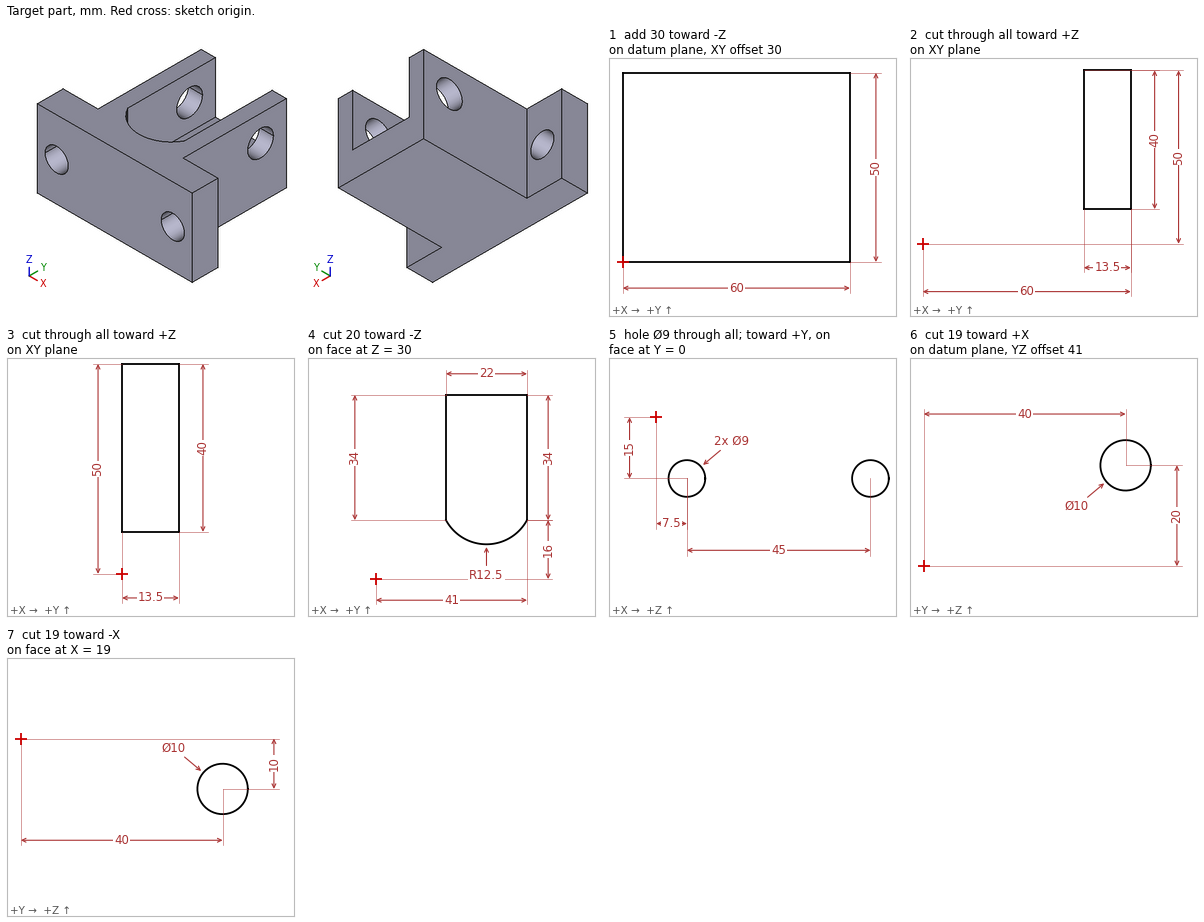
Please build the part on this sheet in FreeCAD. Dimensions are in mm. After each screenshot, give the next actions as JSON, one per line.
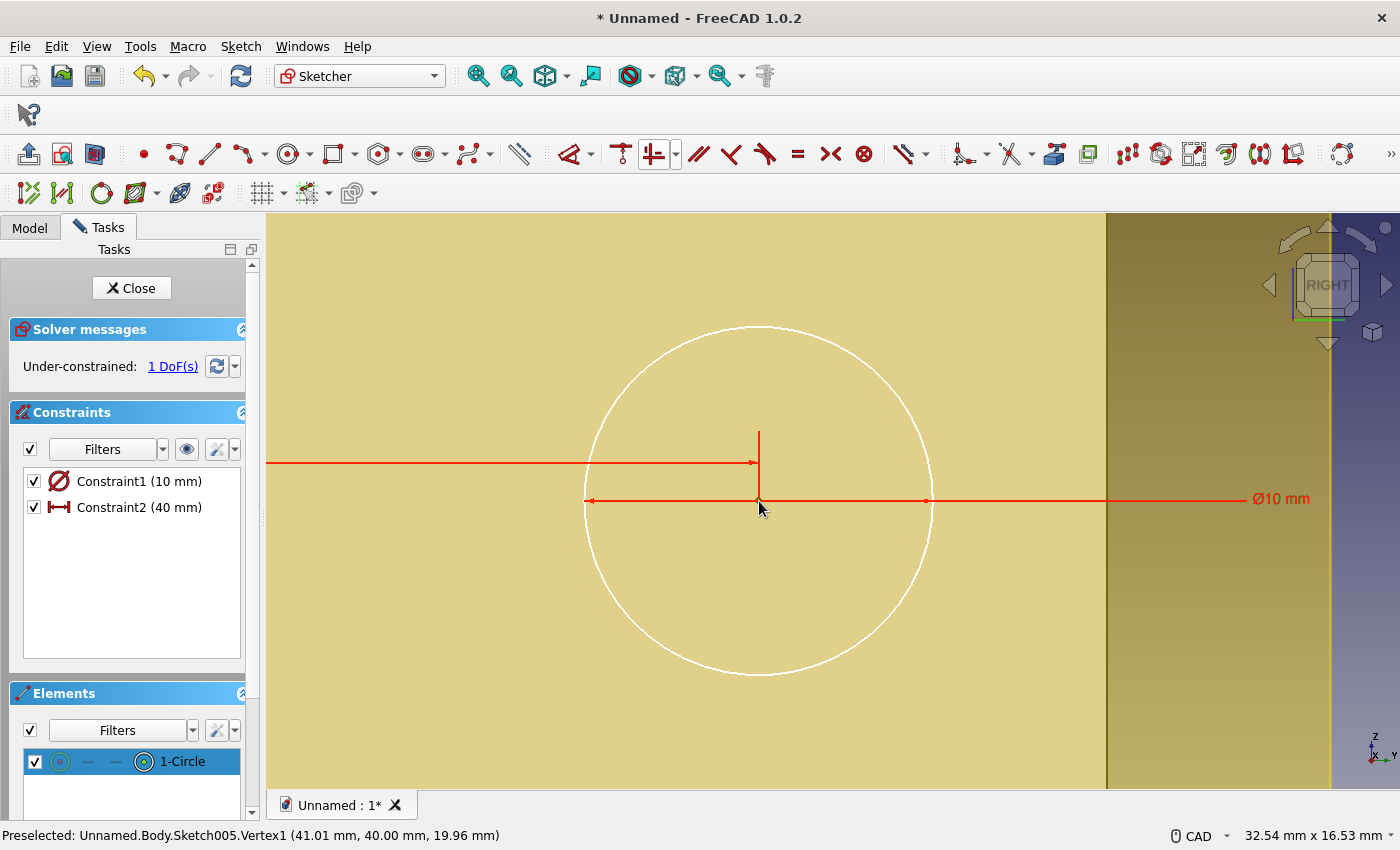
{"action": "key", "text": "i"}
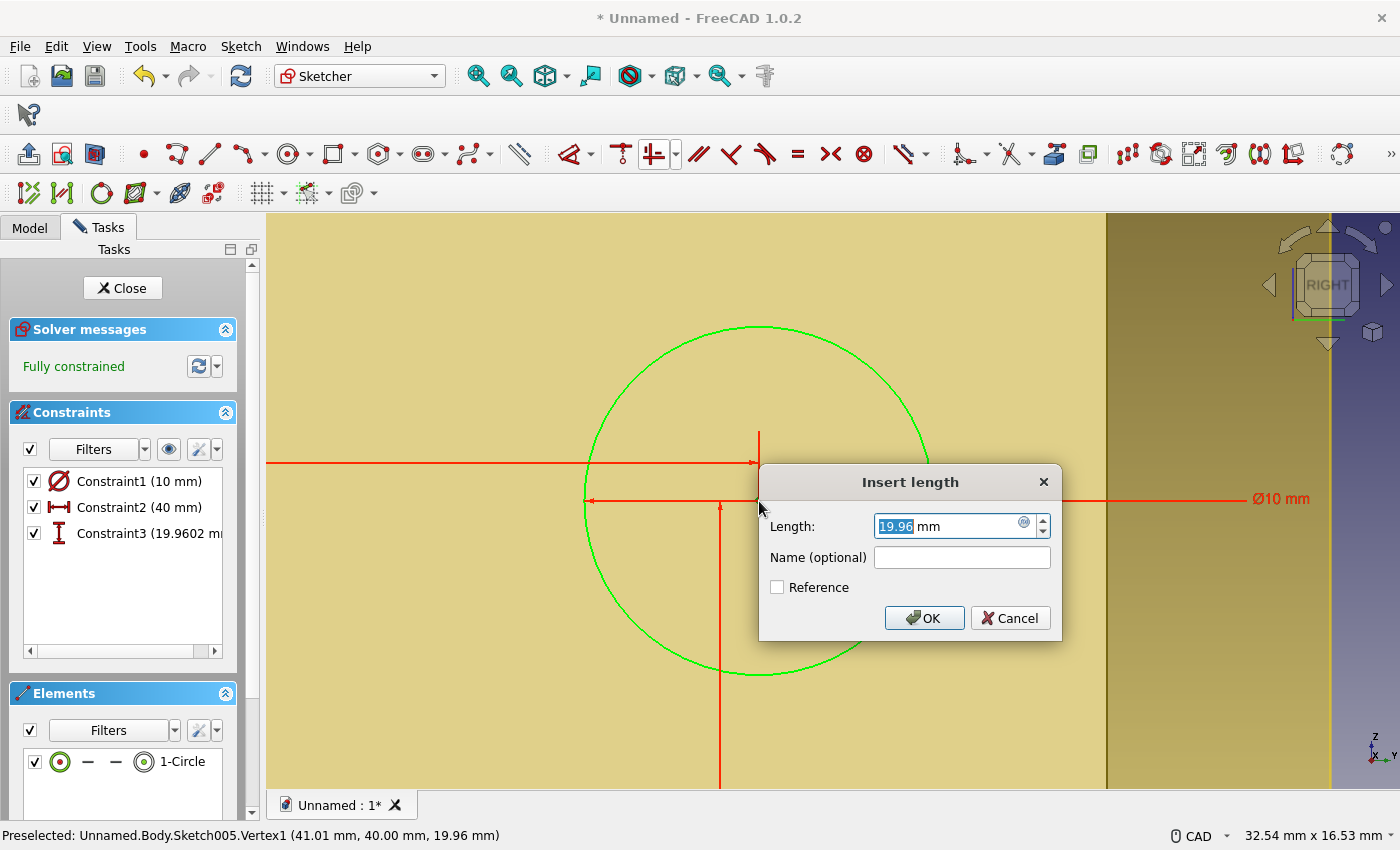
{"action": "type", "text": "20"}
{"action": "key", "text": "Return"}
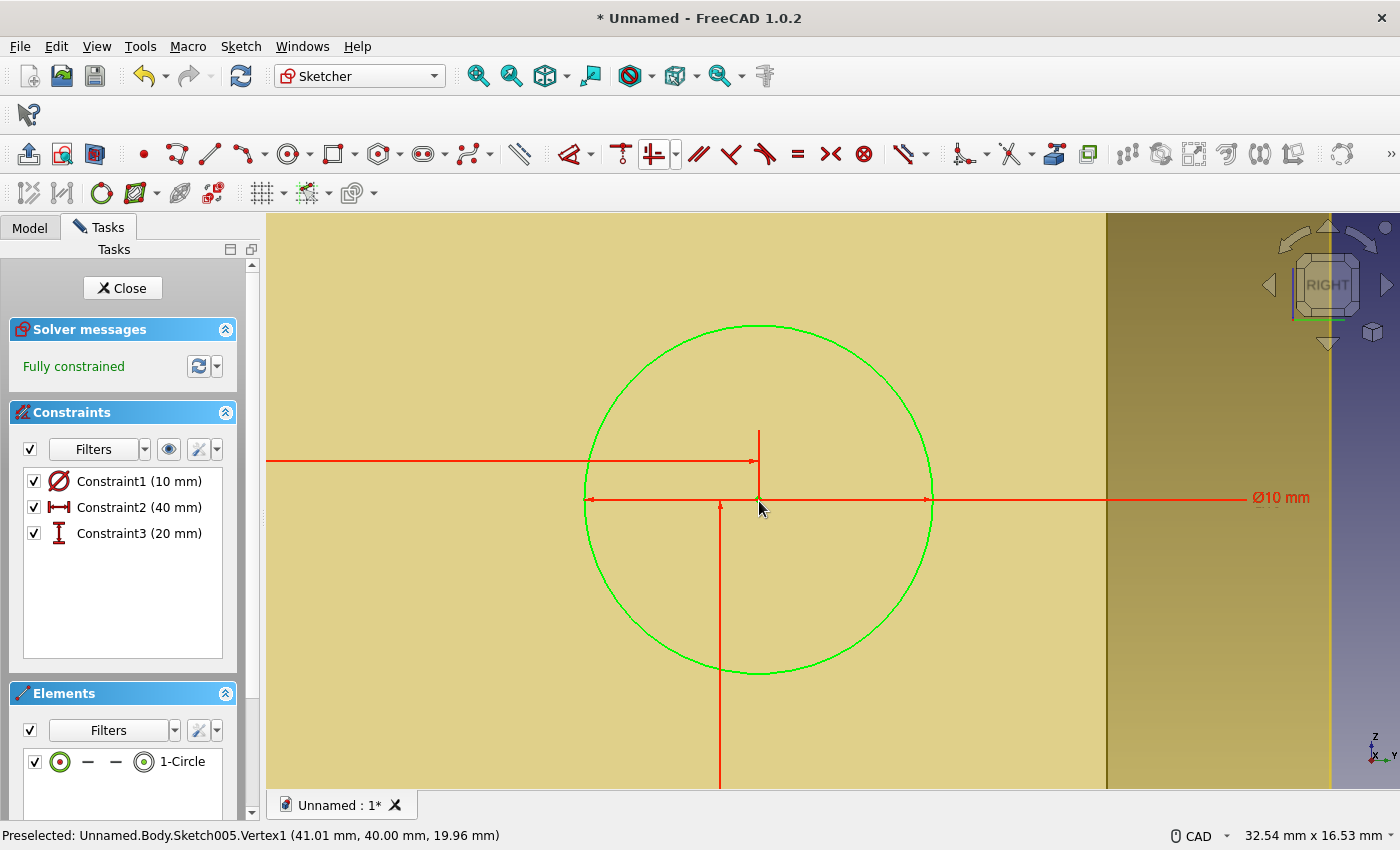
{"action": "left_click", "coordinate": [123, 288]}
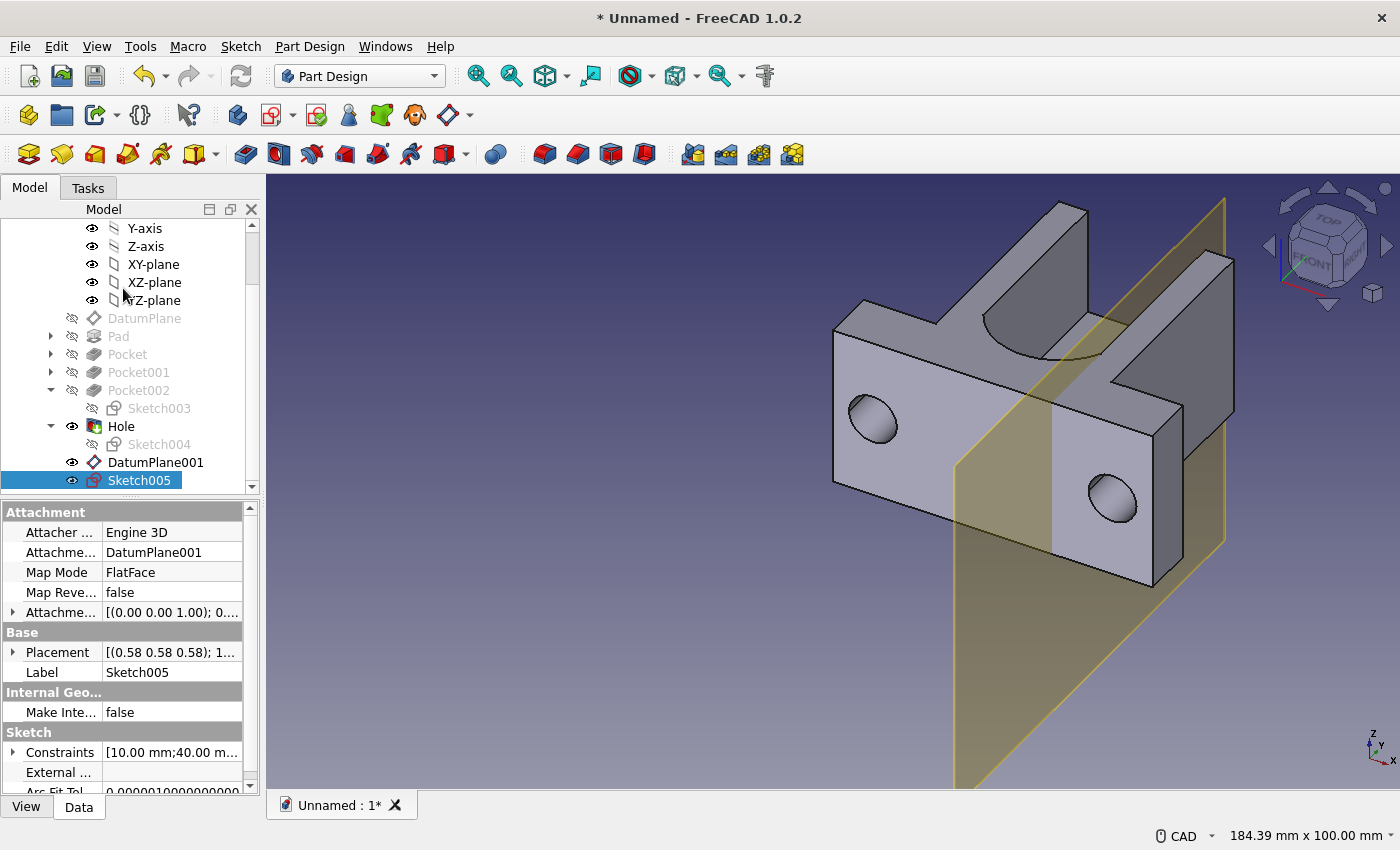
{"action": "left_click", "coordinate": [246, 154]}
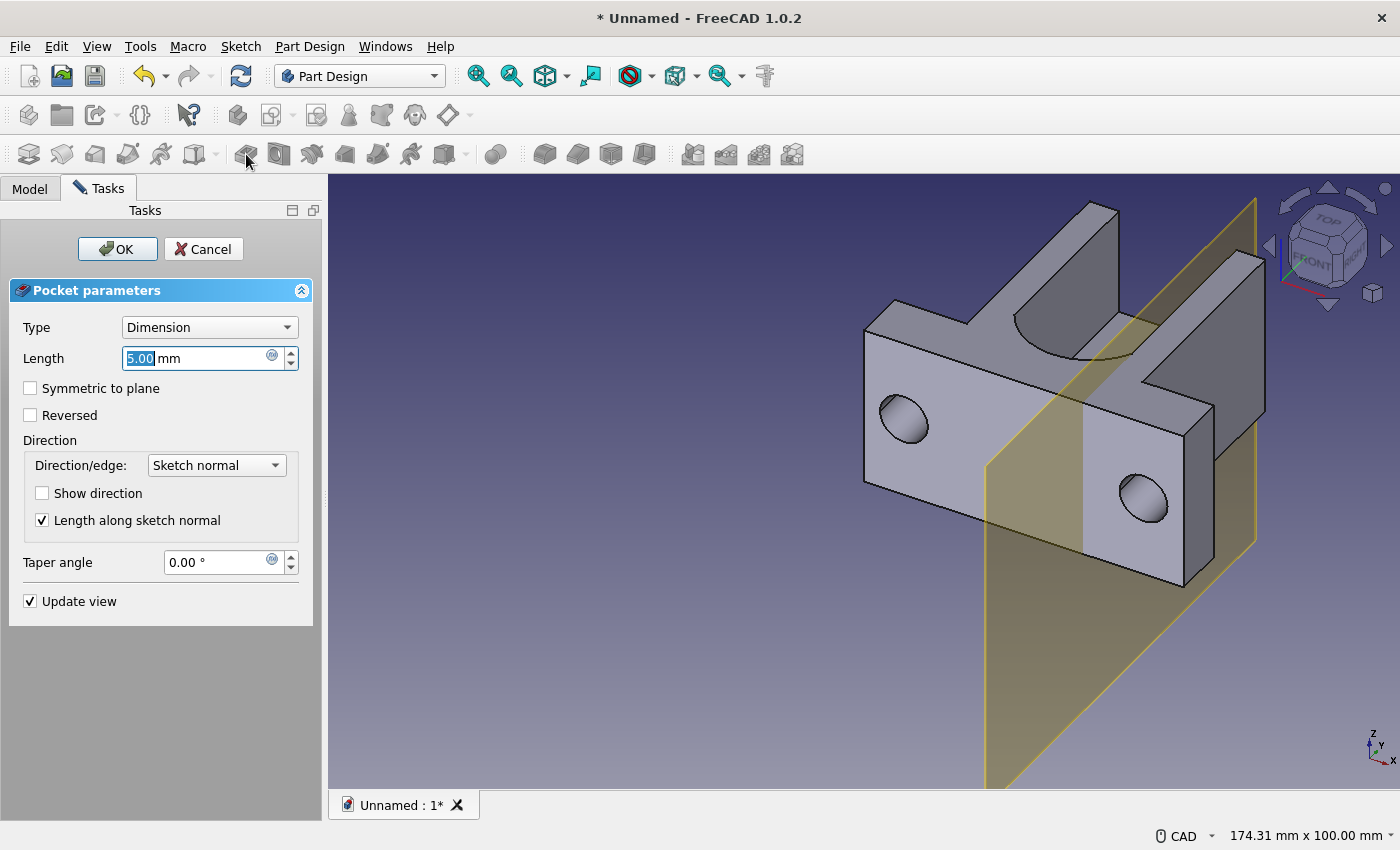
{"action": "type", "text": "19"}
{"action": "key", "text": "Tab"}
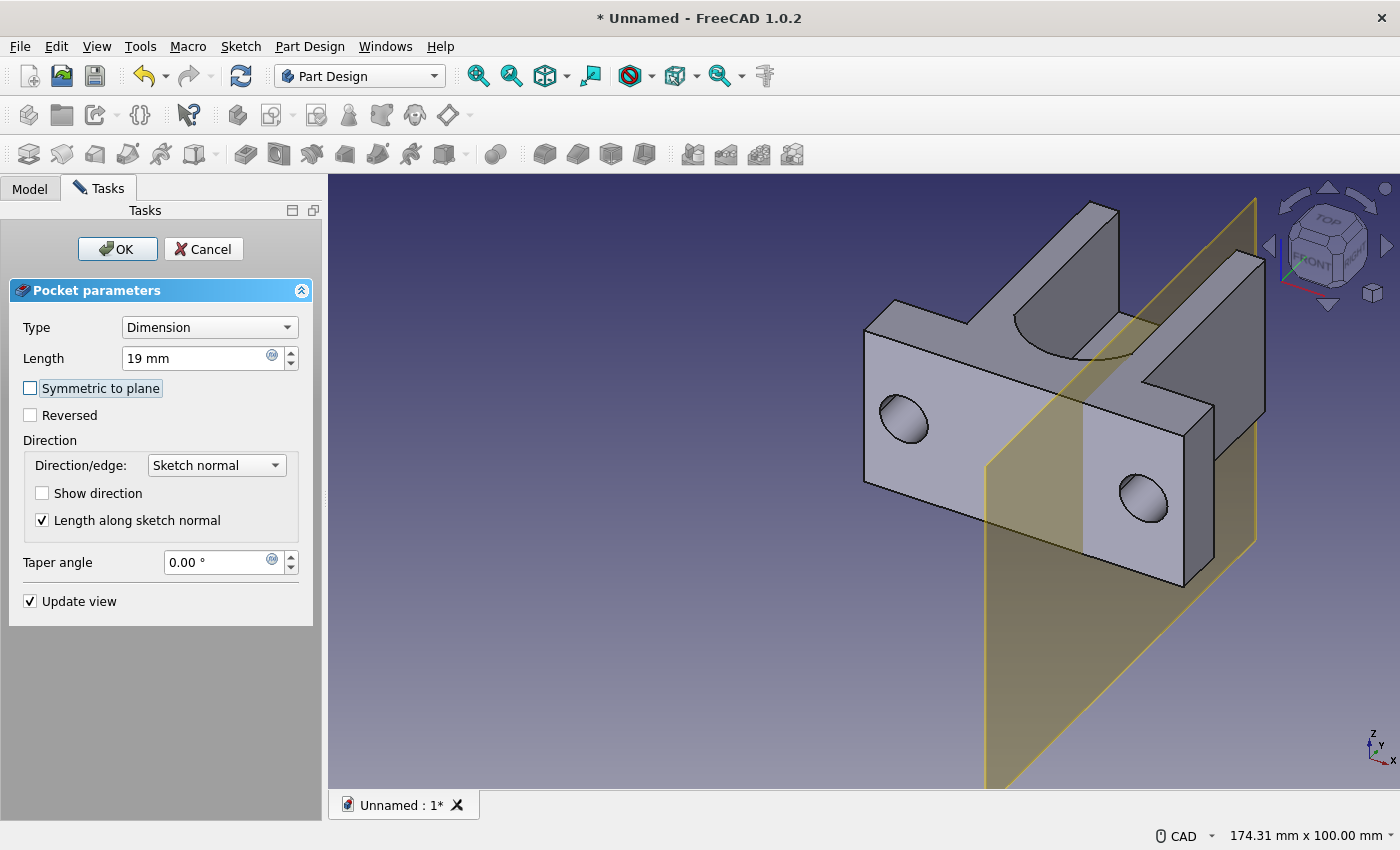
{"action": "left_click", "coordinate": [31, 415]}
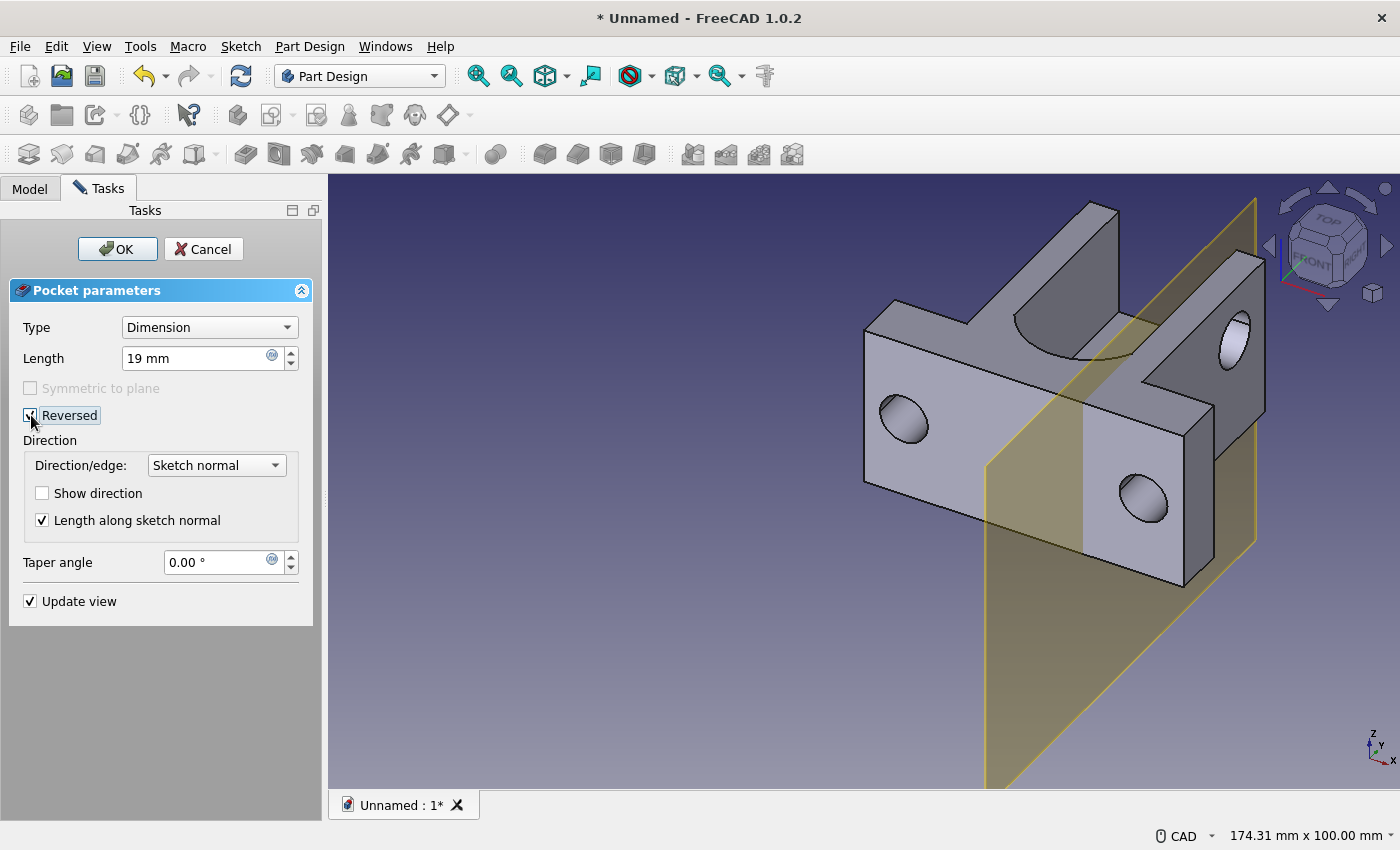
{"action": "left_click", "coordinate": [118, 249]}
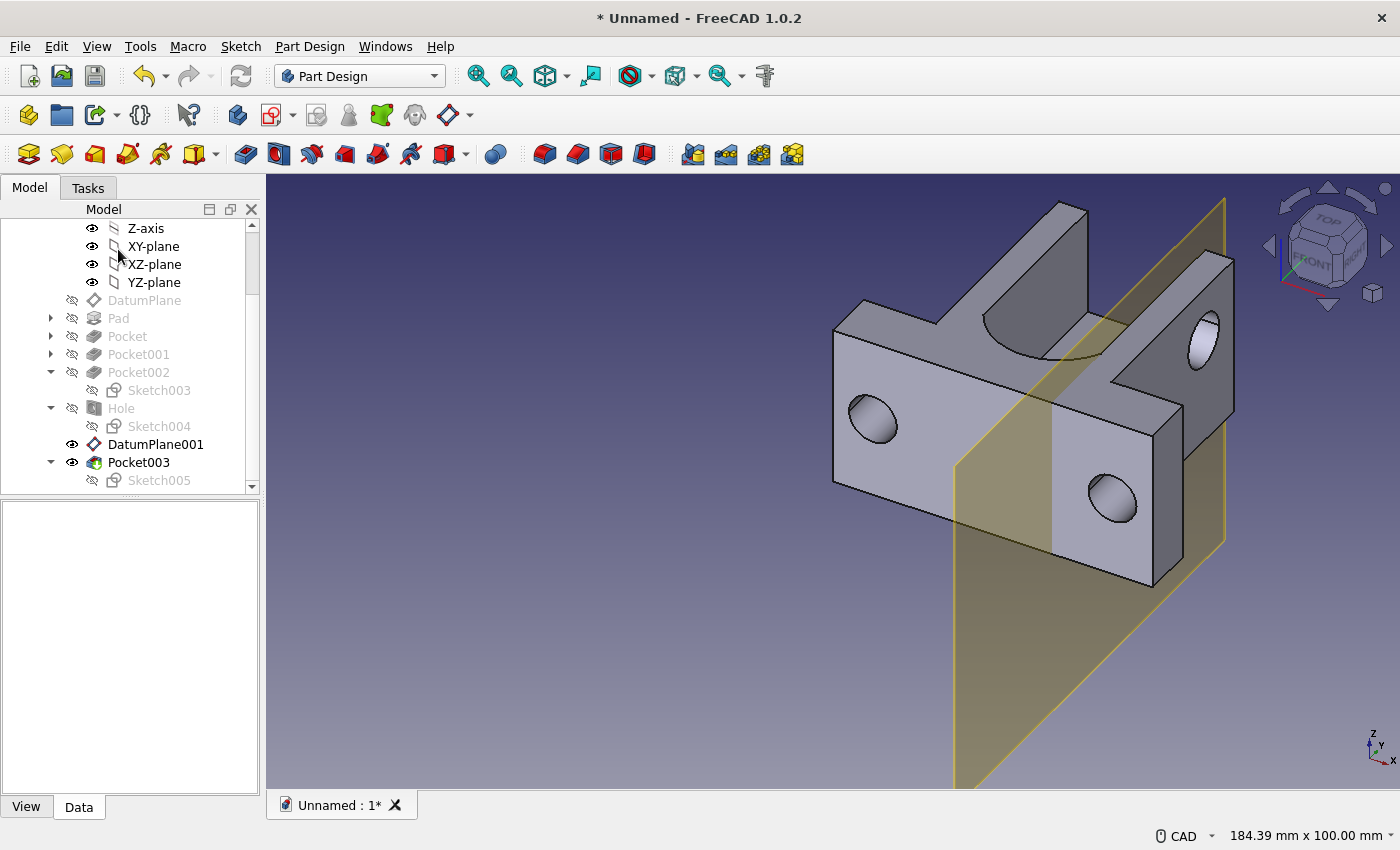
{"action": "left_click", "coordinate": [117, 444]}
{"action": "key", "text": "space"}